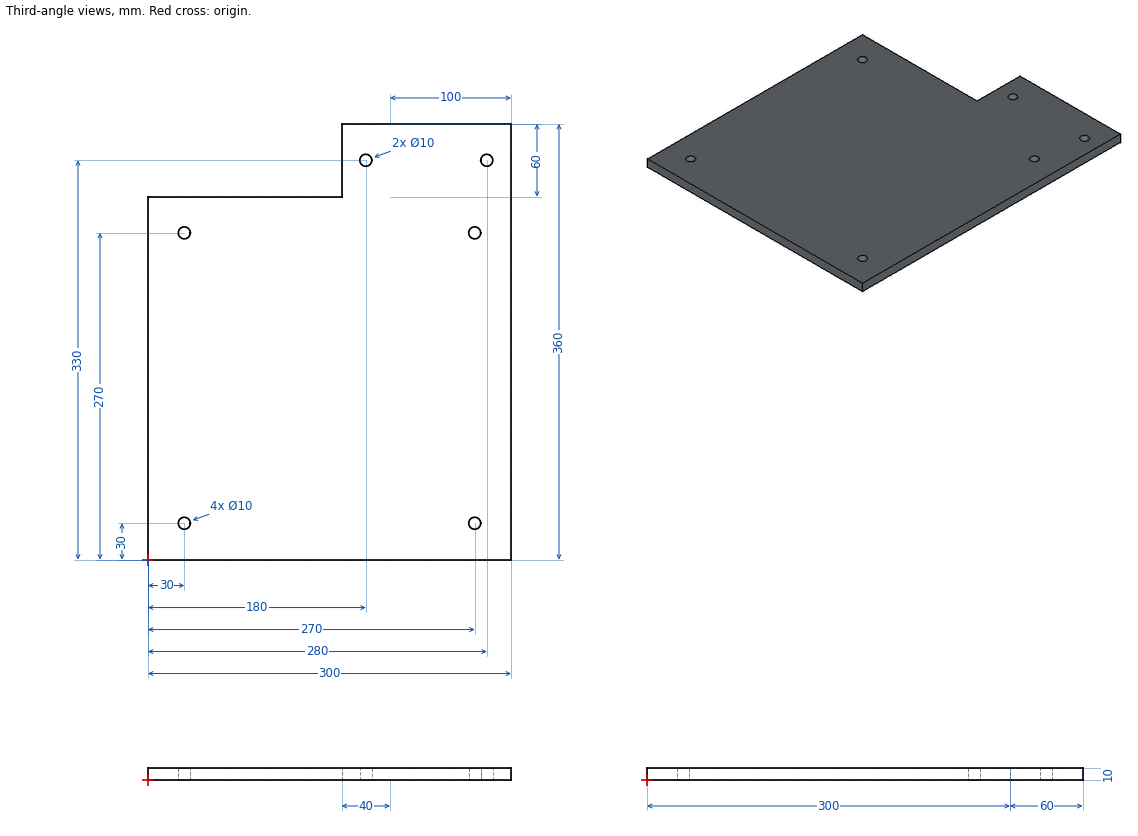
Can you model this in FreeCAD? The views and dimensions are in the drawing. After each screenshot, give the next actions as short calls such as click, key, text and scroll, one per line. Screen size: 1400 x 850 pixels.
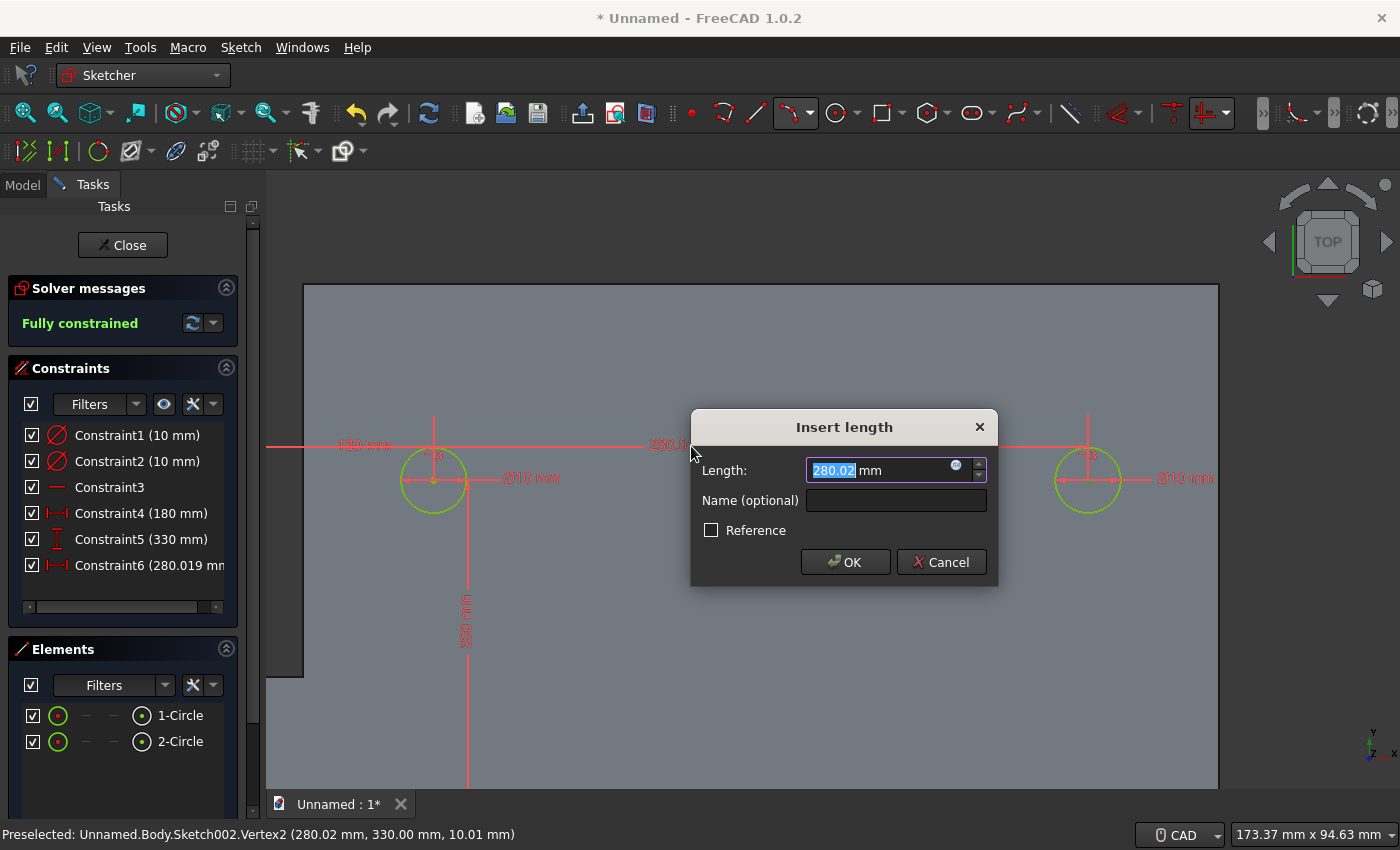
text(280)
key(Return)
key(Escape)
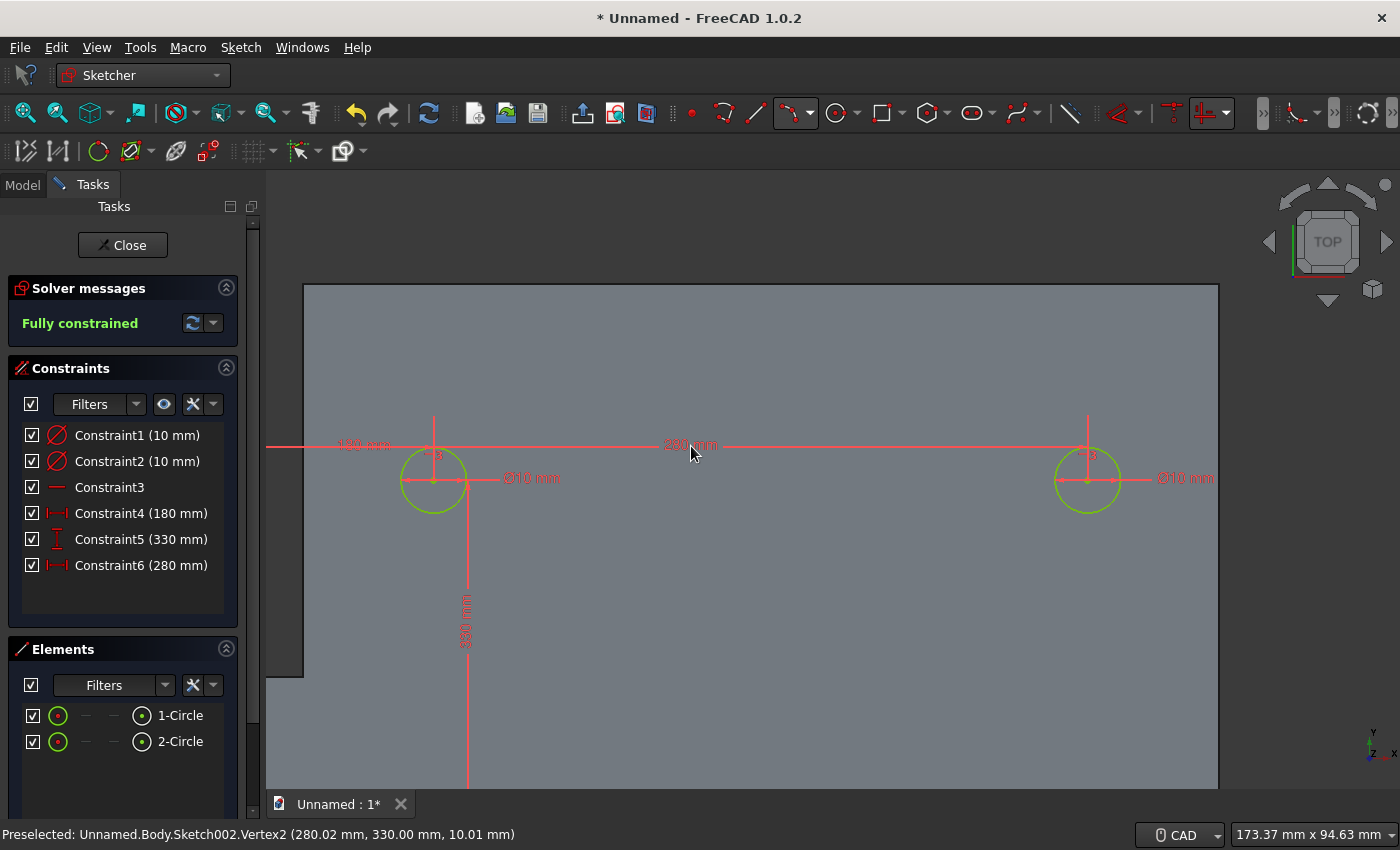
click(123, 245)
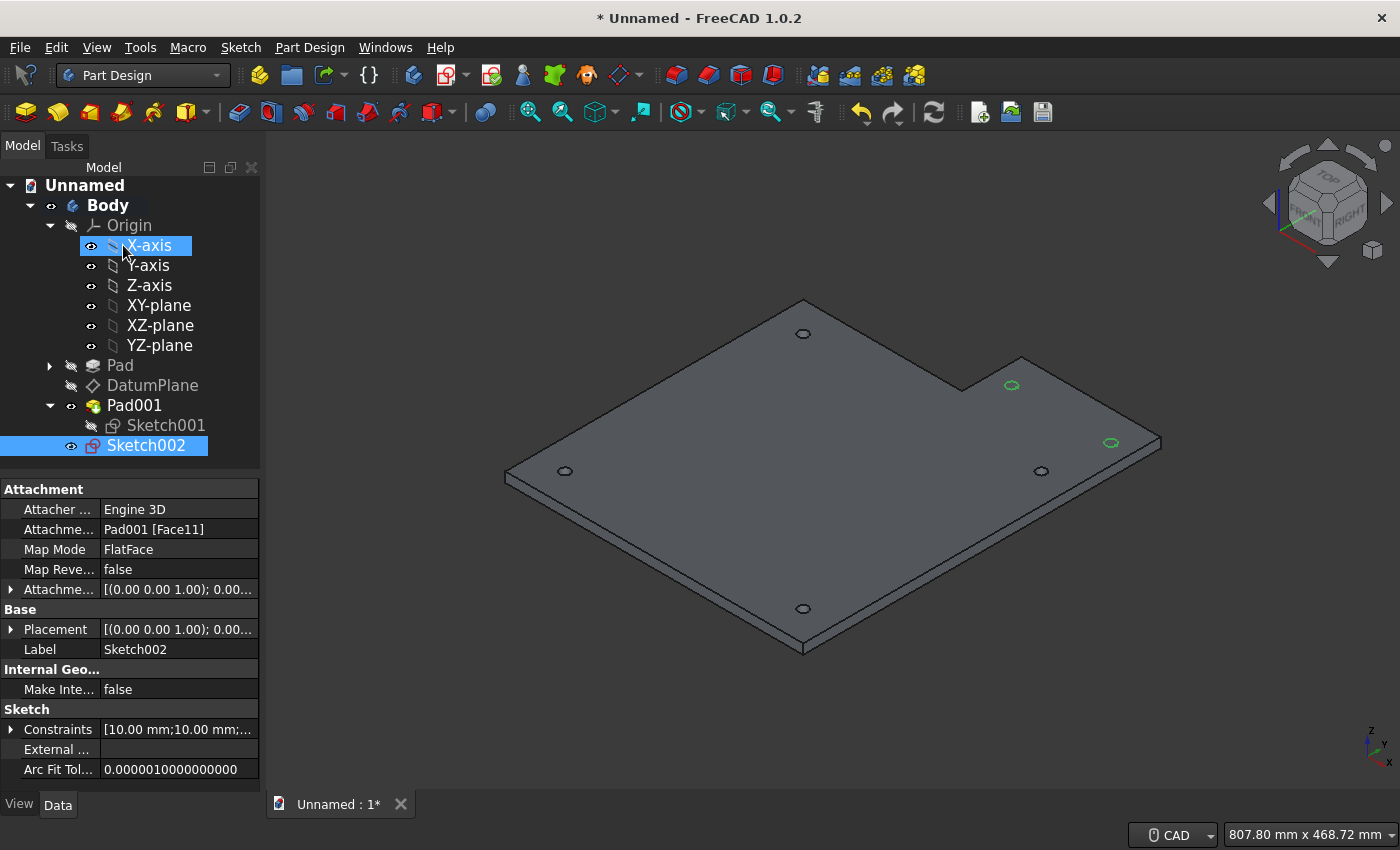
click(240, 112)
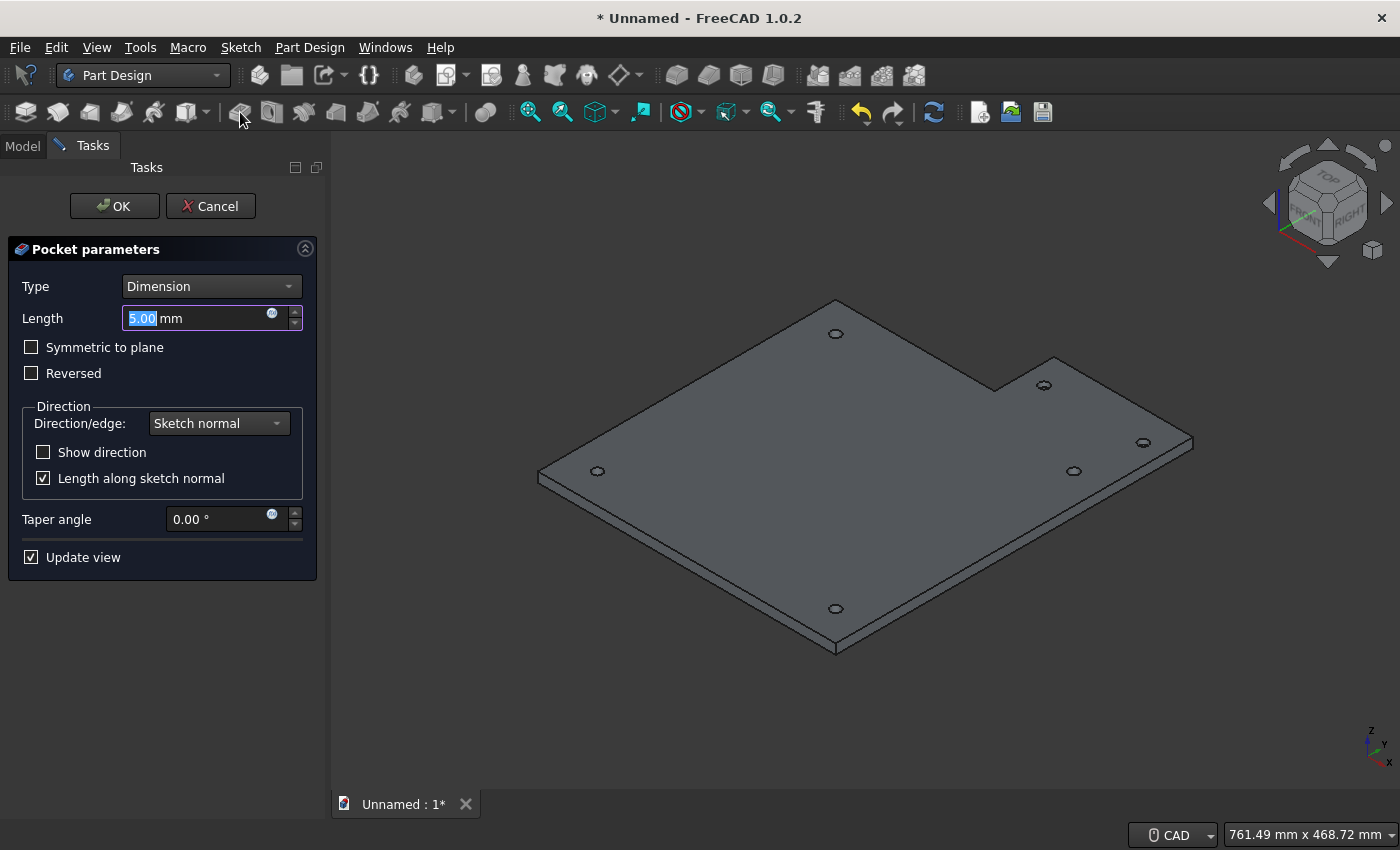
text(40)
key(Tab)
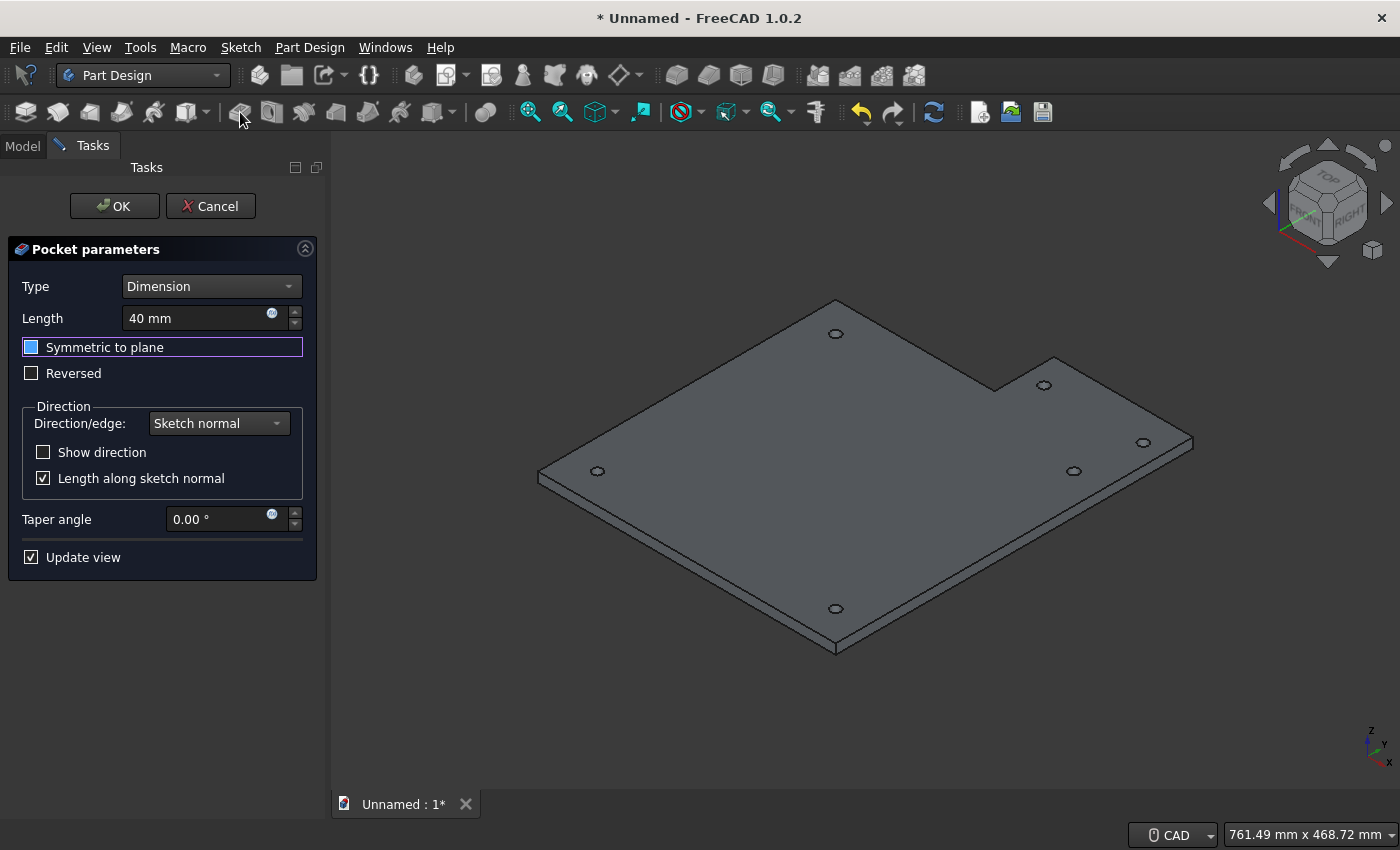
click(115, 206)